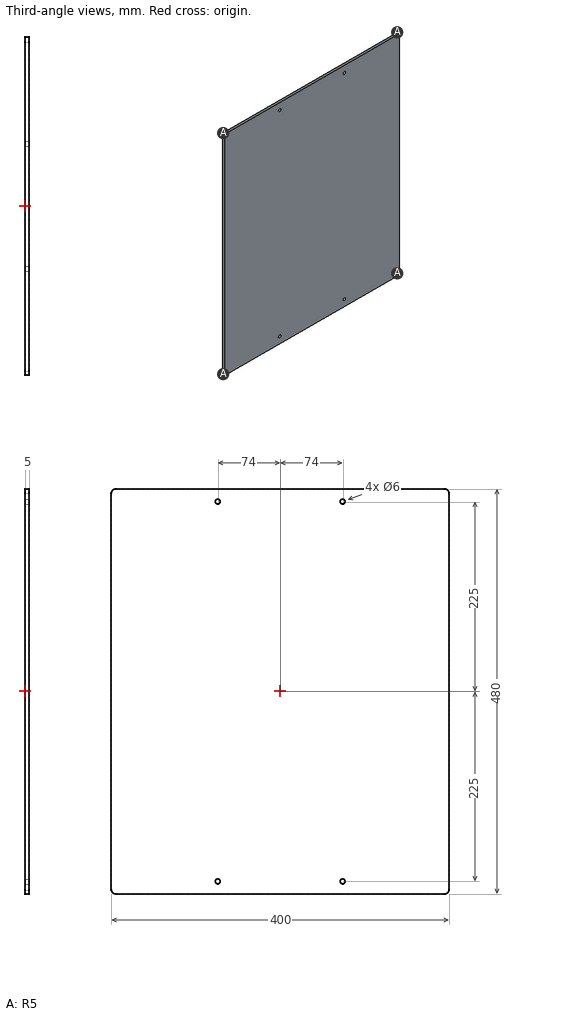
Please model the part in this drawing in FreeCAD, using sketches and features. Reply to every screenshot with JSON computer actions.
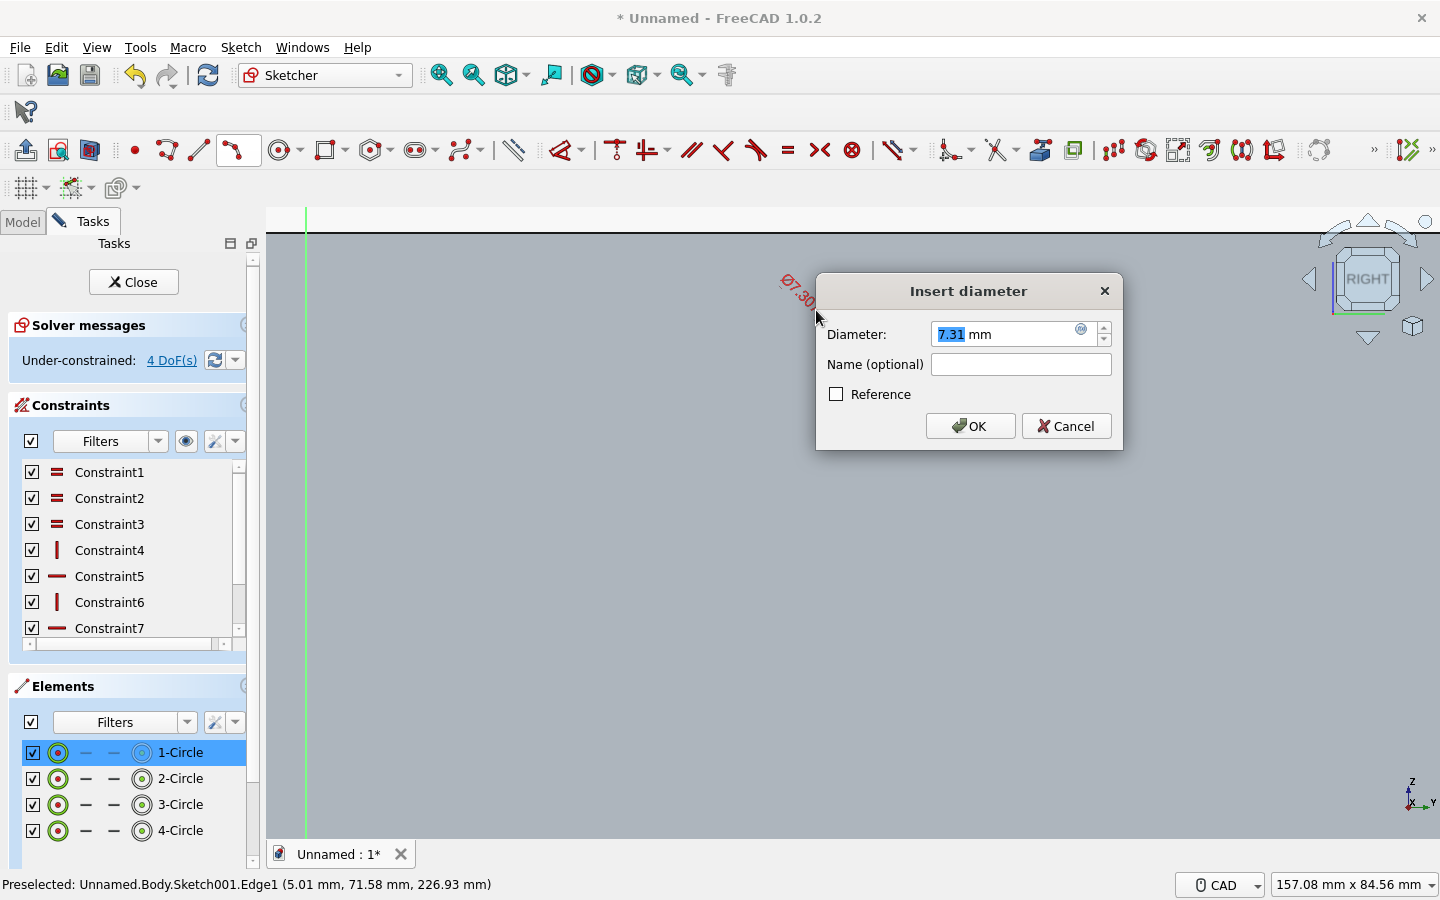
{"action": "type", "text": "6"}
{"action": "key", "text": "Return"}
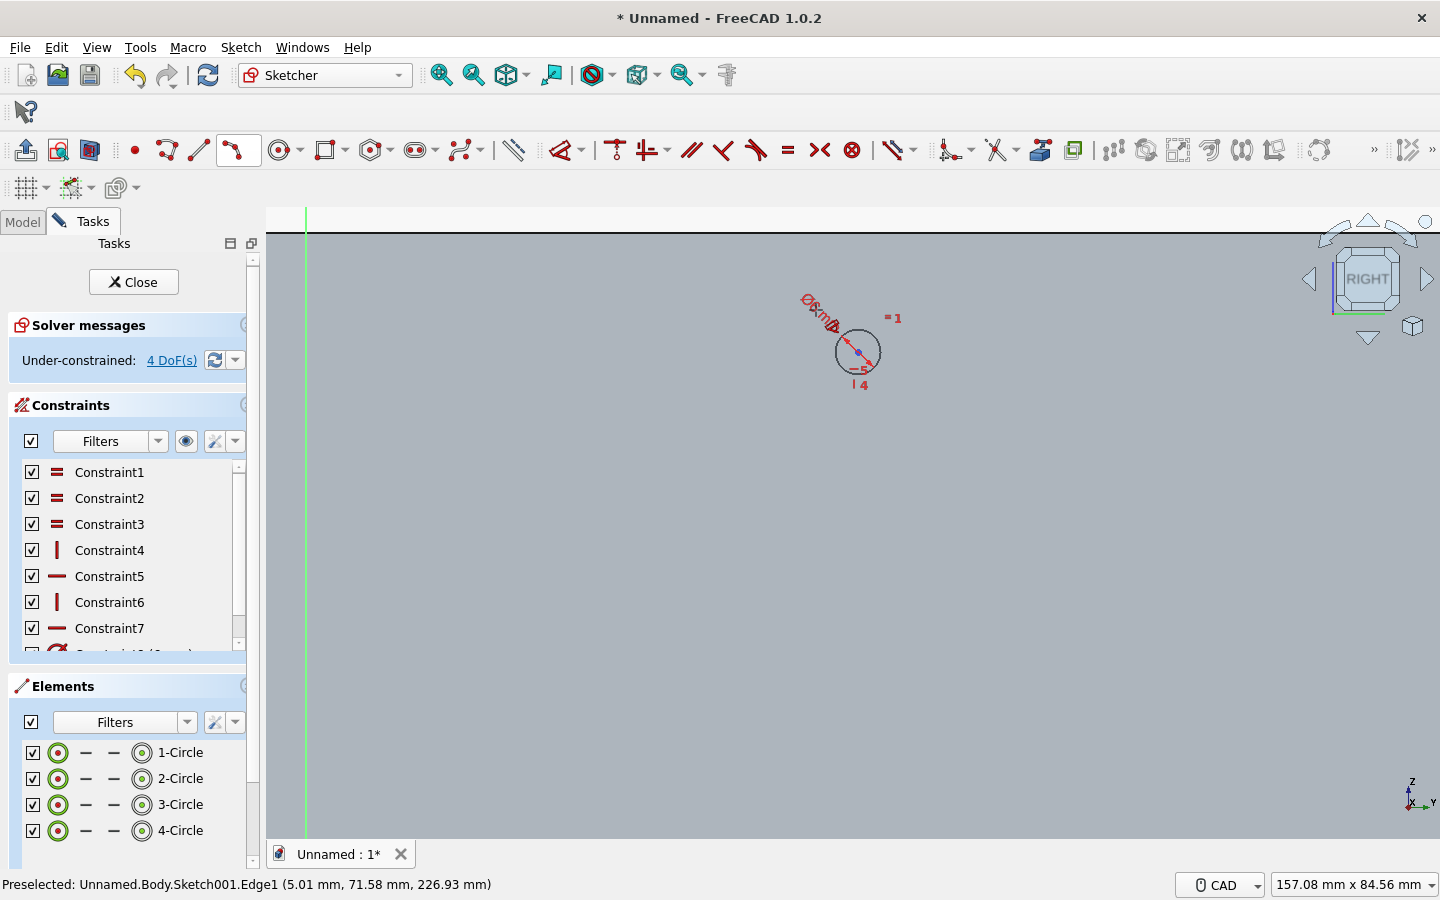
{"action": "scroll", "coordinate": [844, 336], "scroll_direction": "down", "scroll_amount": 11}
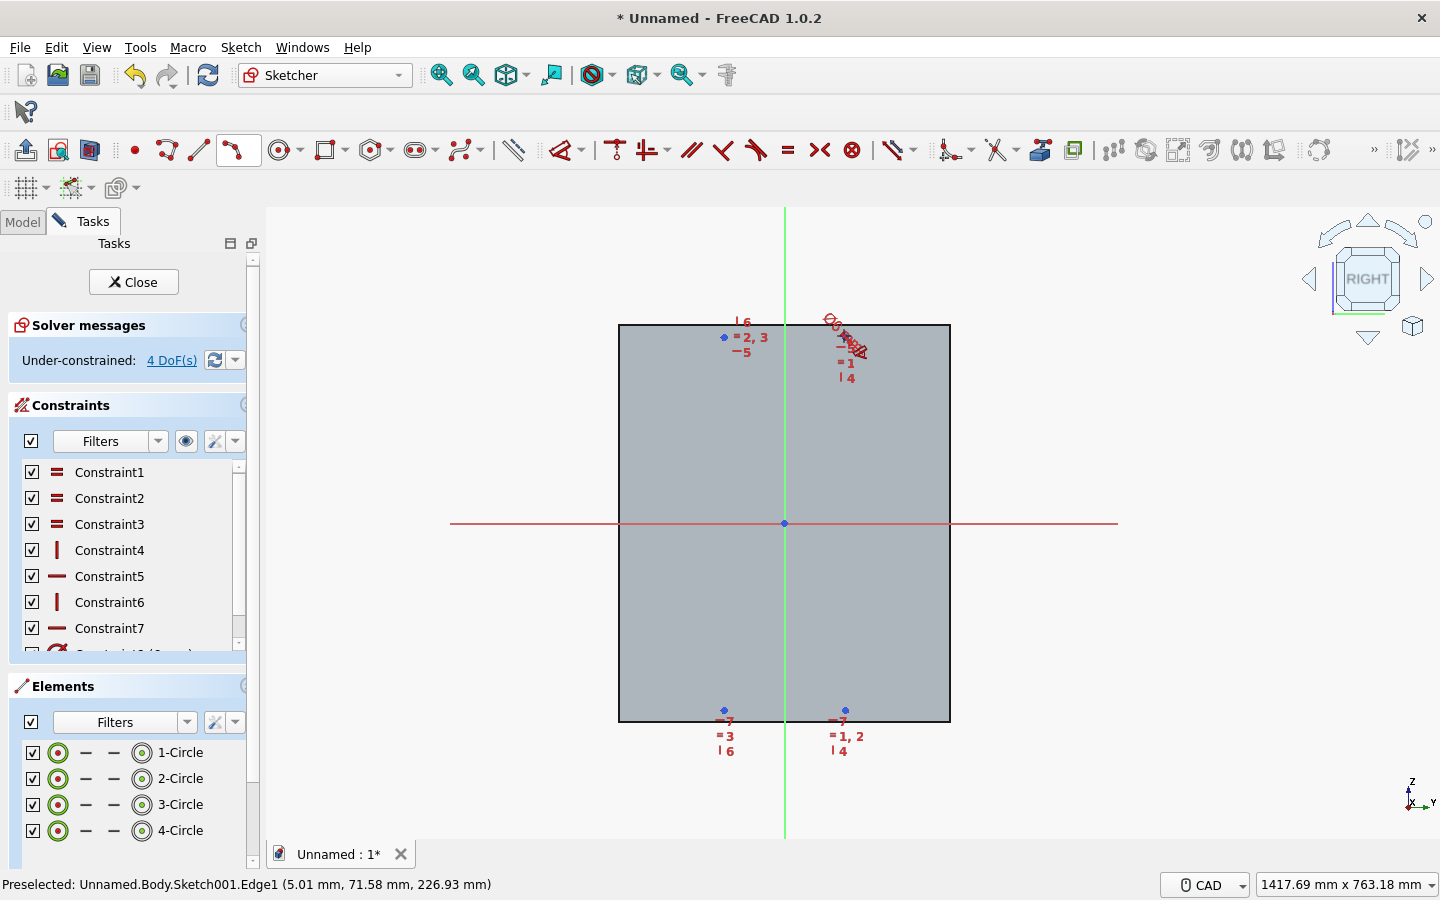
{"action": "left_click", "coordinate": [846, 338]}
{"action": "left_click", "coordinate": [815, 304]}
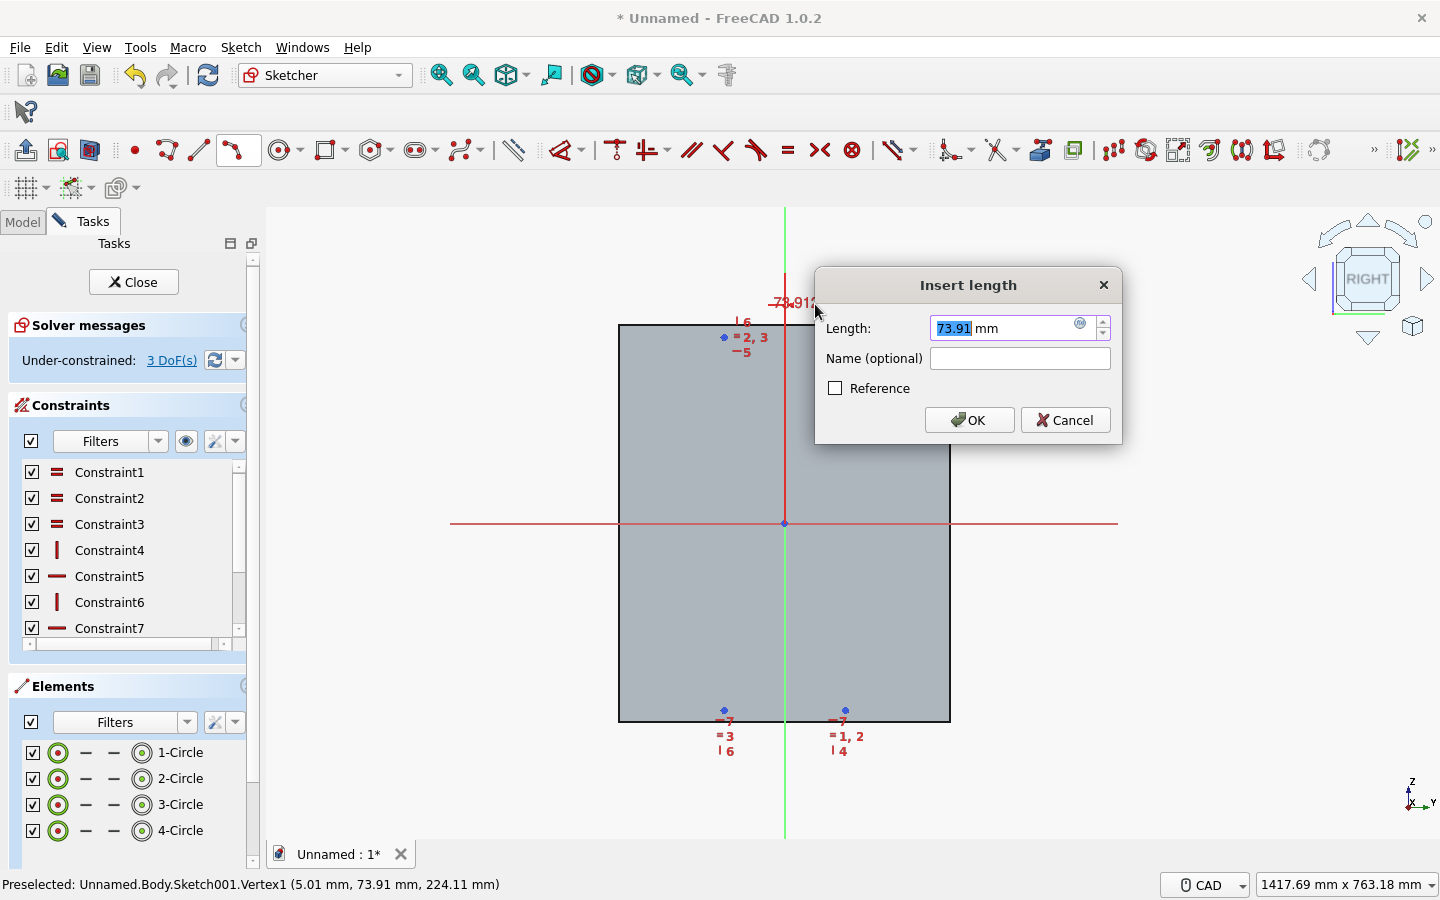
{"action": "type", "text": "74"}
{"action": "key", "text": "Return"}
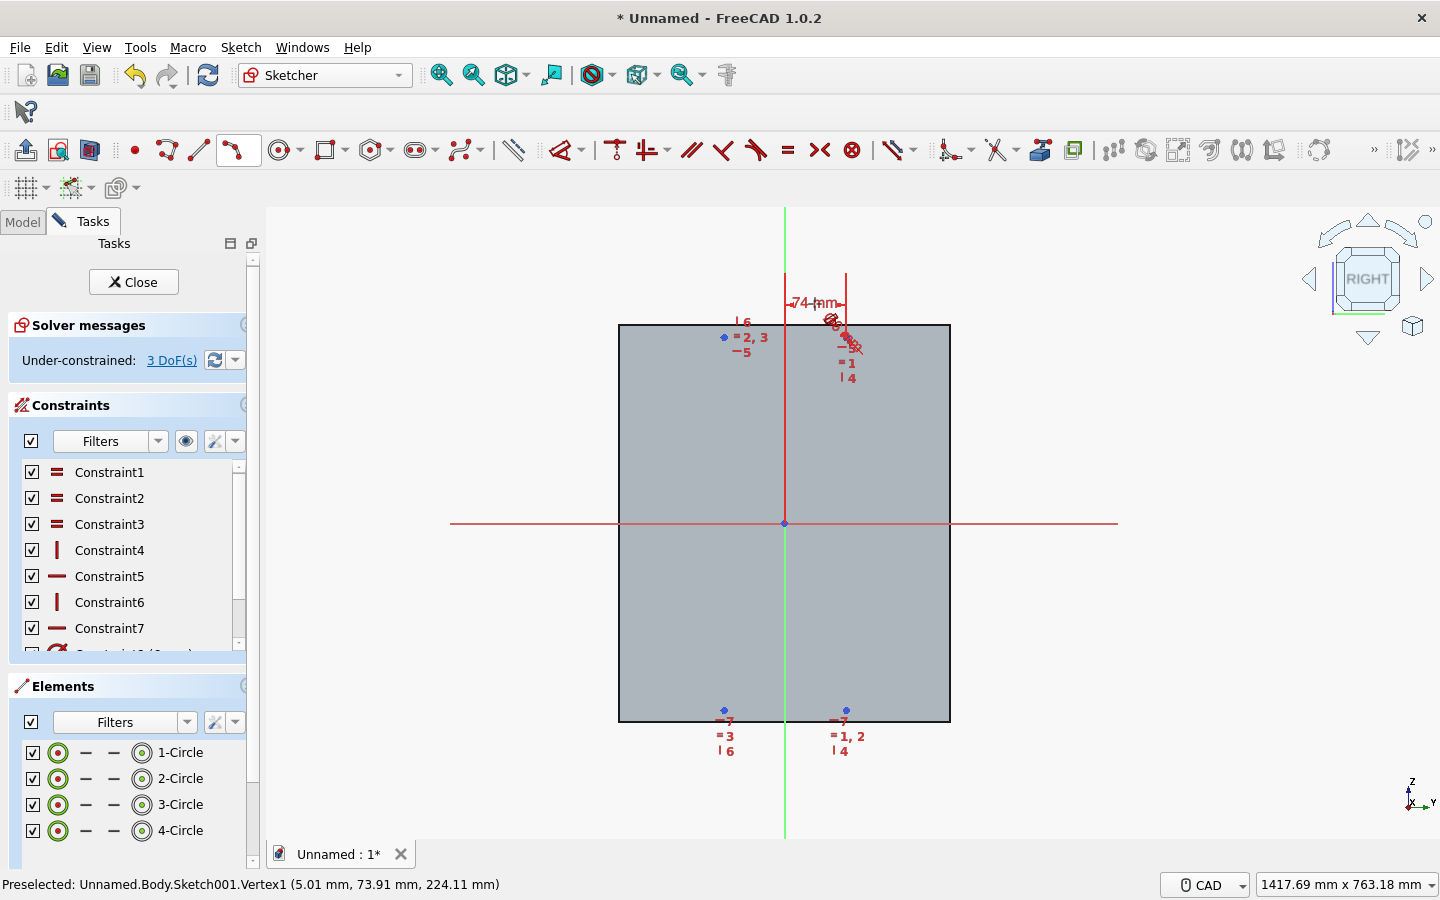
{"action": "left_click", "coordinate": [724, 338]}
{"action": "left_click", "coordinate": [740, 304]}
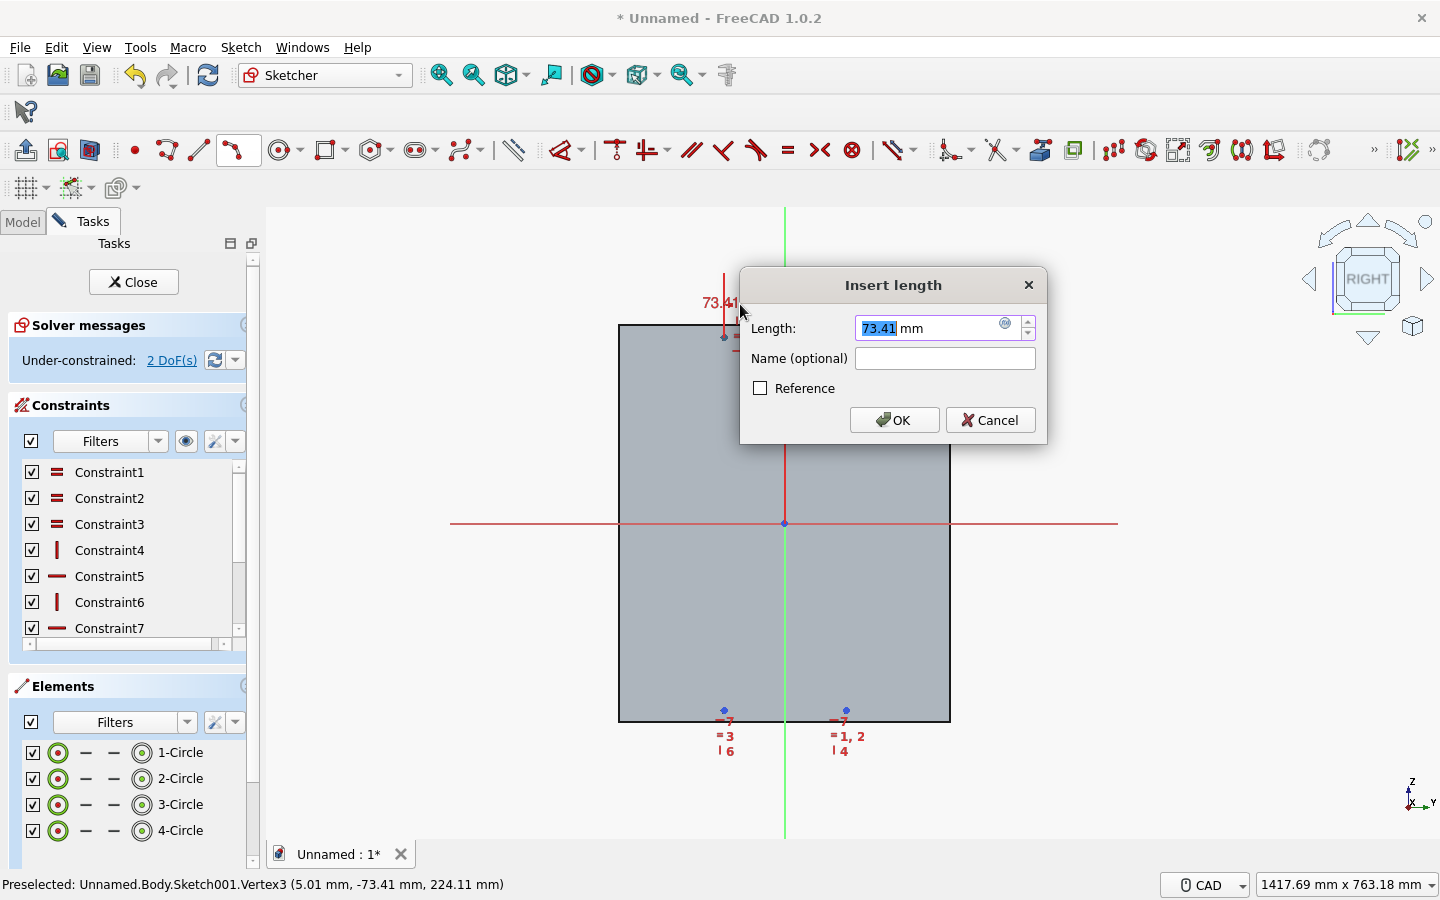
{"action": "type", "text": "74"}
{"action": "key", "text": "Return"}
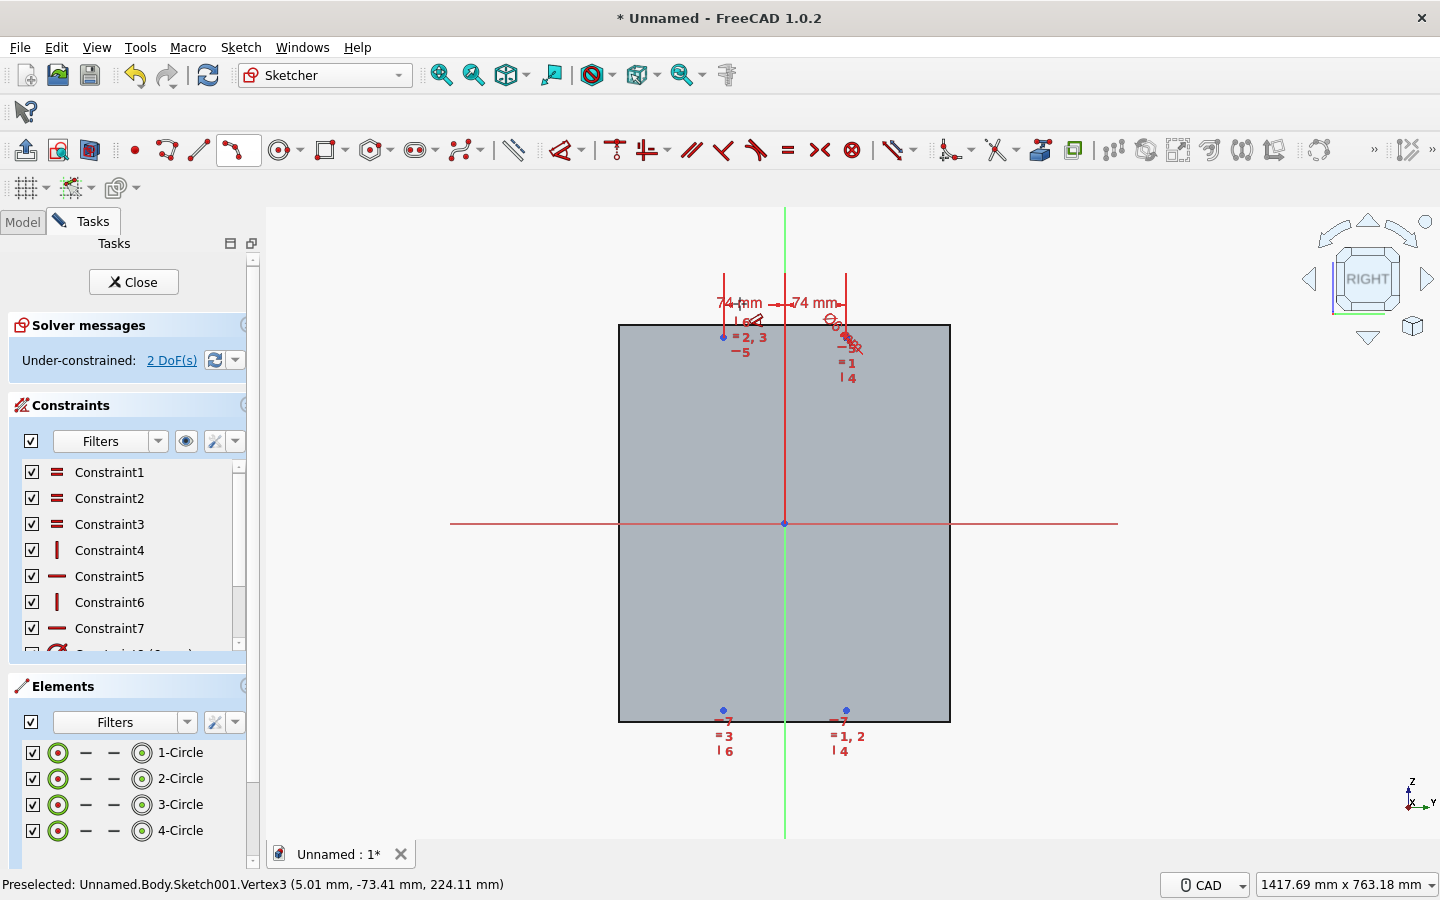
{"action": "left_click", "coordinate": [846, 338]}
{"action": "left_click", "coordinate": [880, 431]}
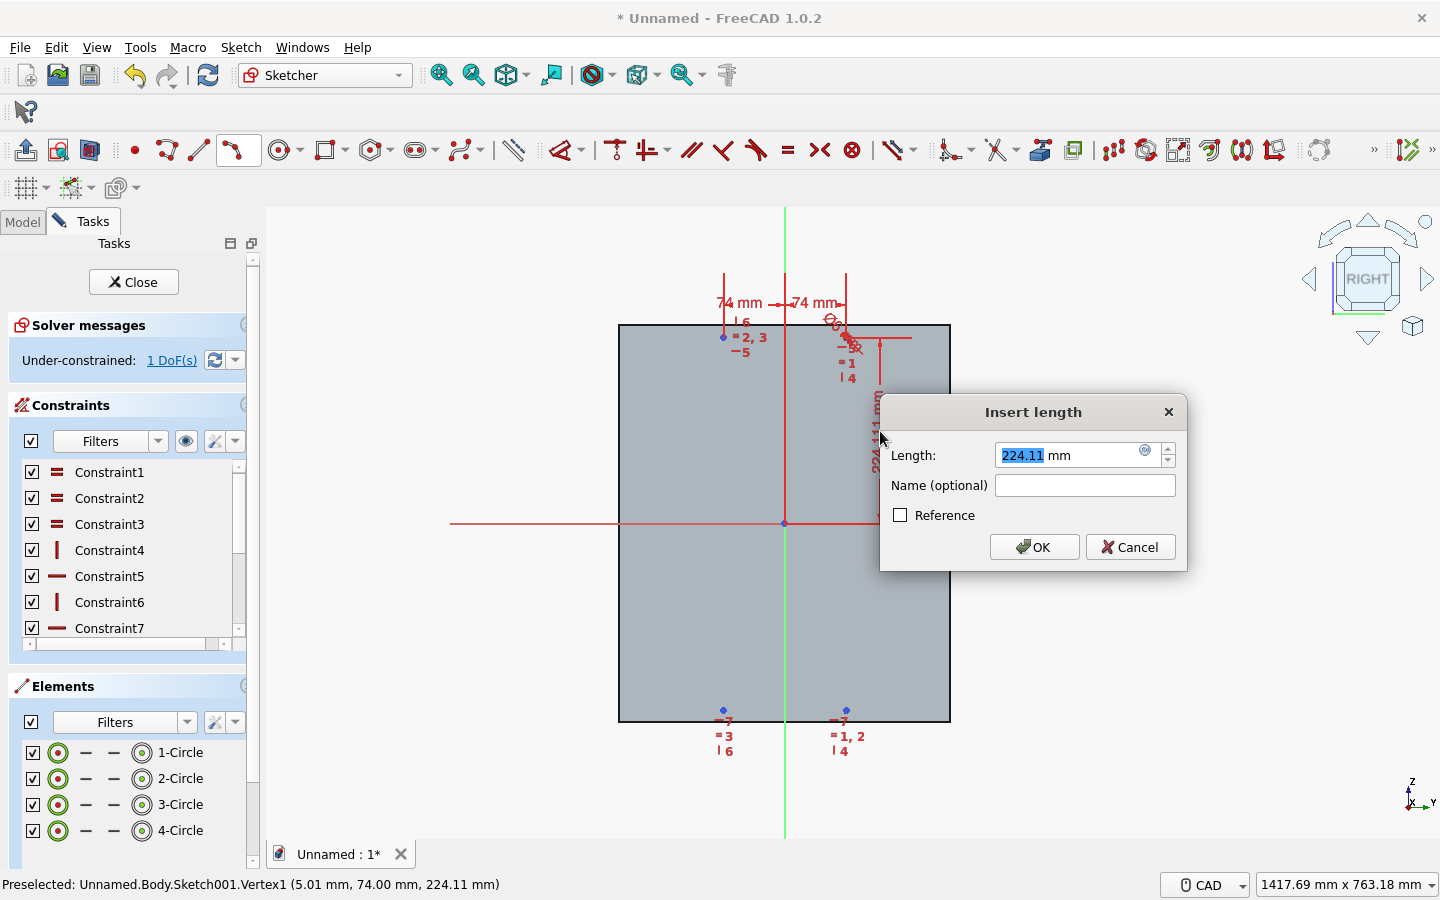
{"action": "type", "text": "225"}
{"action": "key", "text": "Return"}